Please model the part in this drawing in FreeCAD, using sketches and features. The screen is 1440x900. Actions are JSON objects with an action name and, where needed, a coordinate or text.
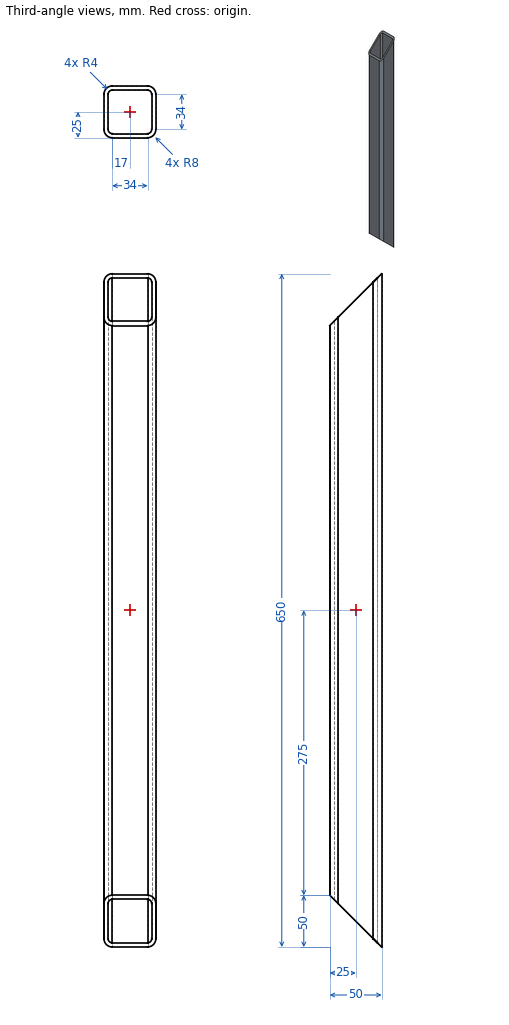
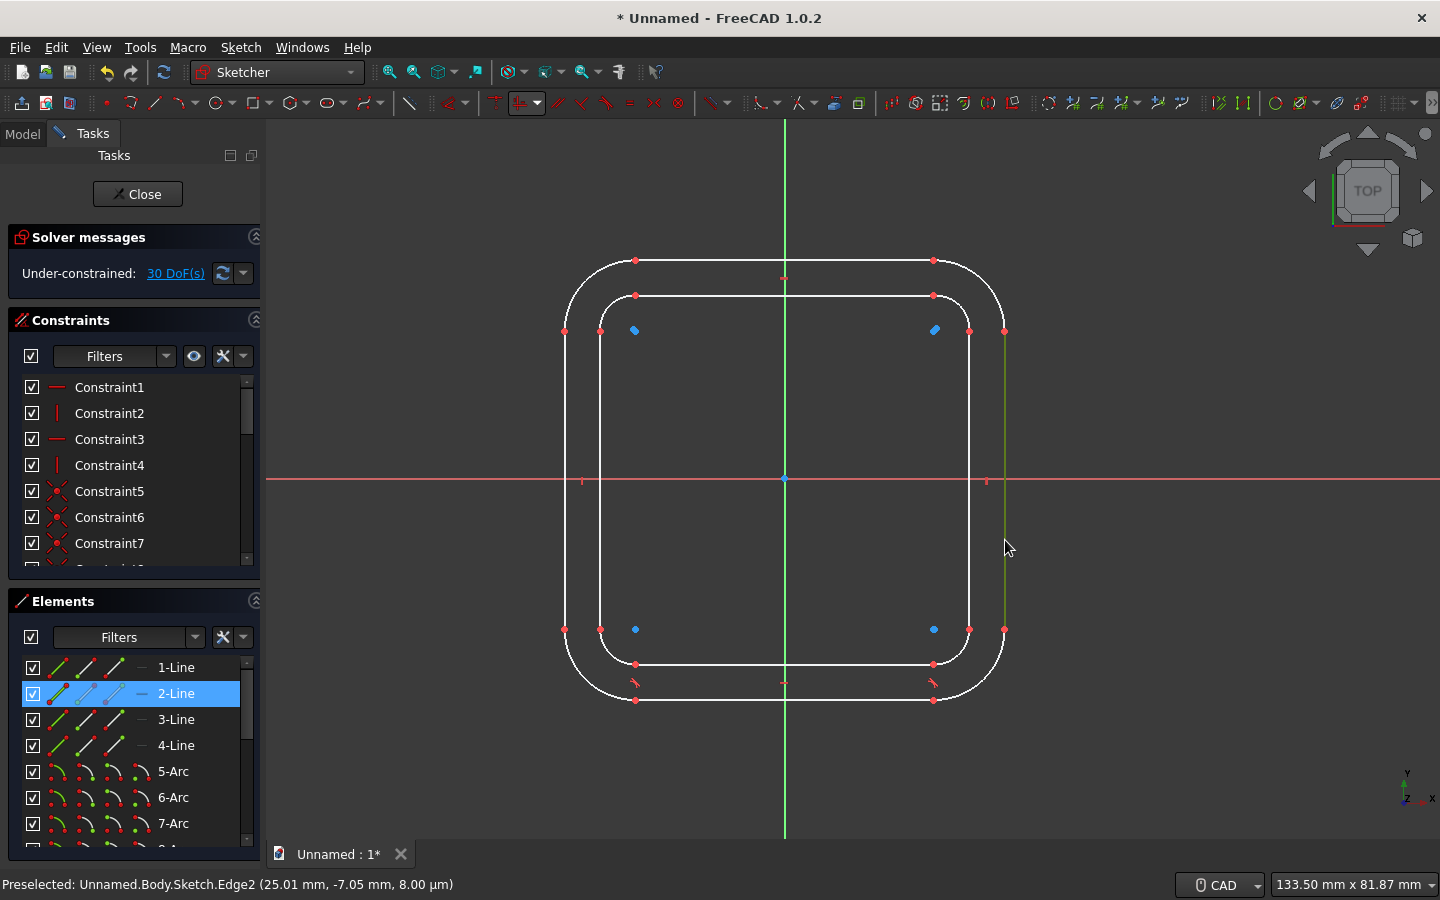
{"action": "left_click", "coordinate": [966, 692]}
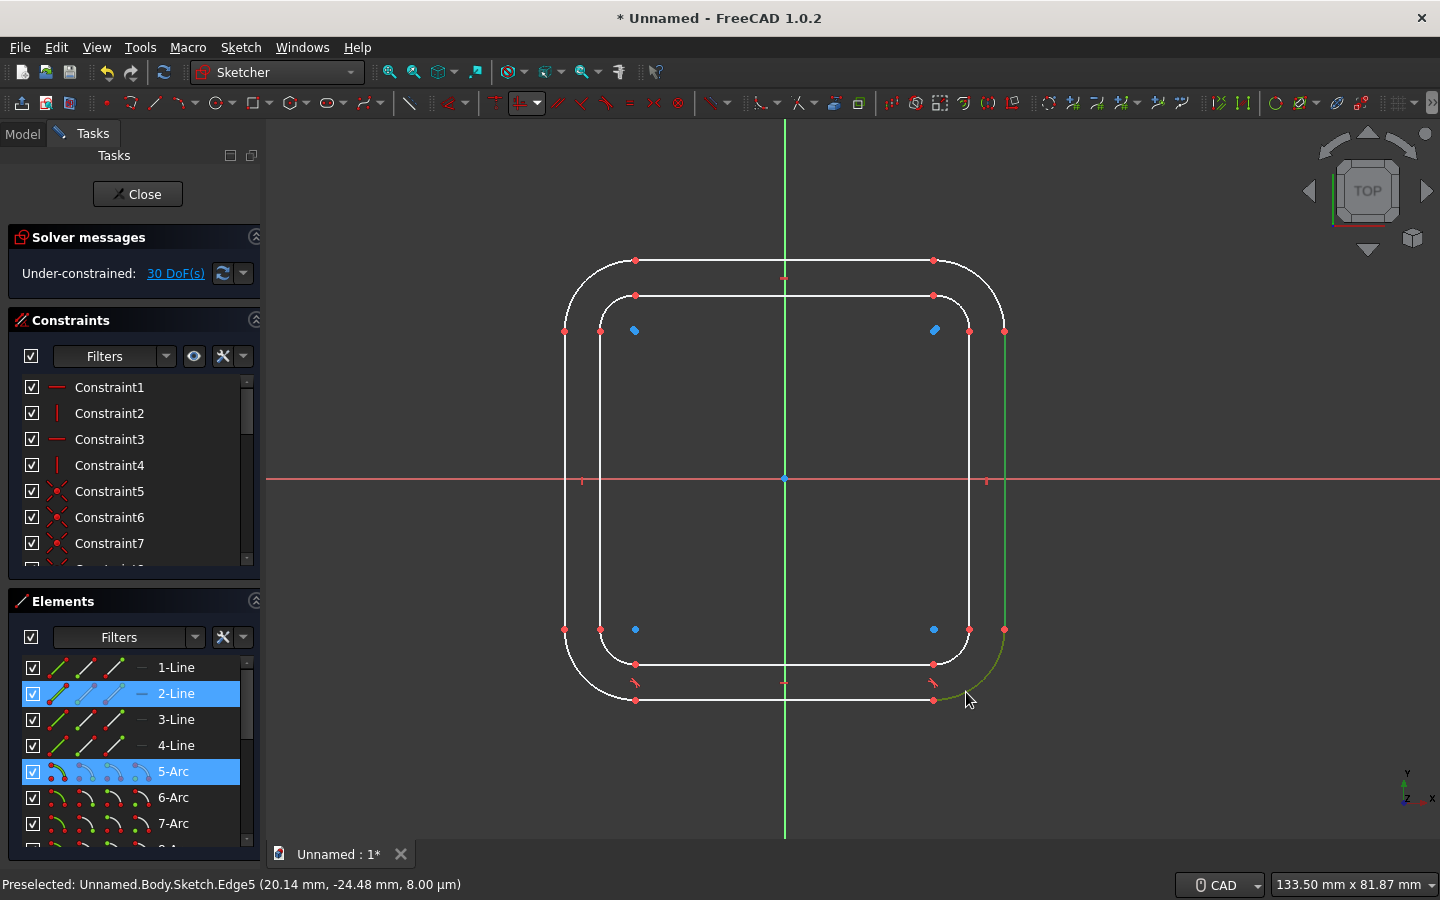
{"action": "left_click", "coordinate": [606, 104]}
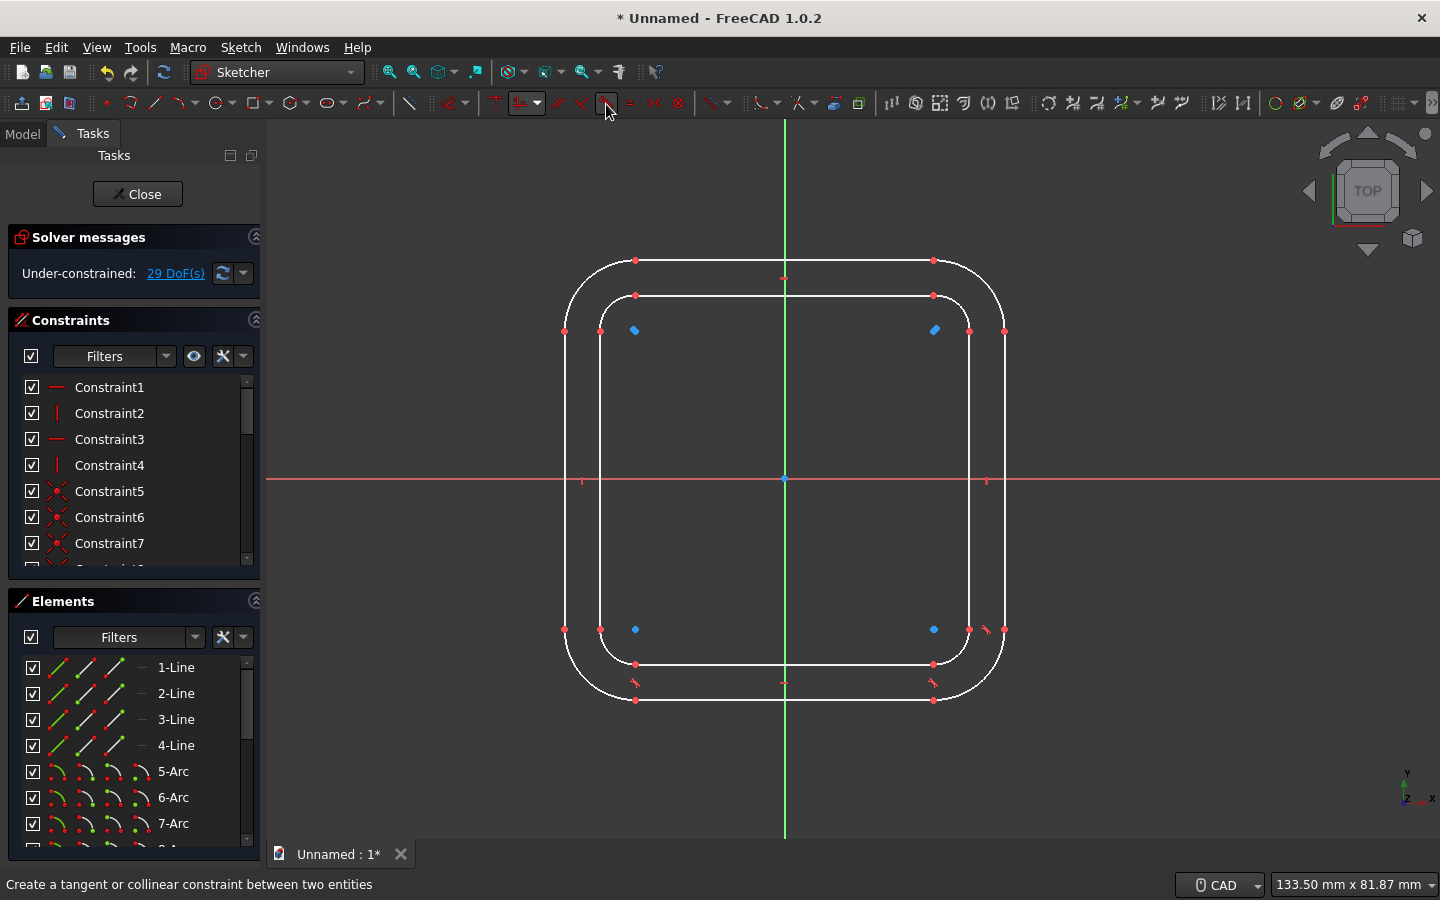
{"action": "left_click", "coordinate": [1005, 540]}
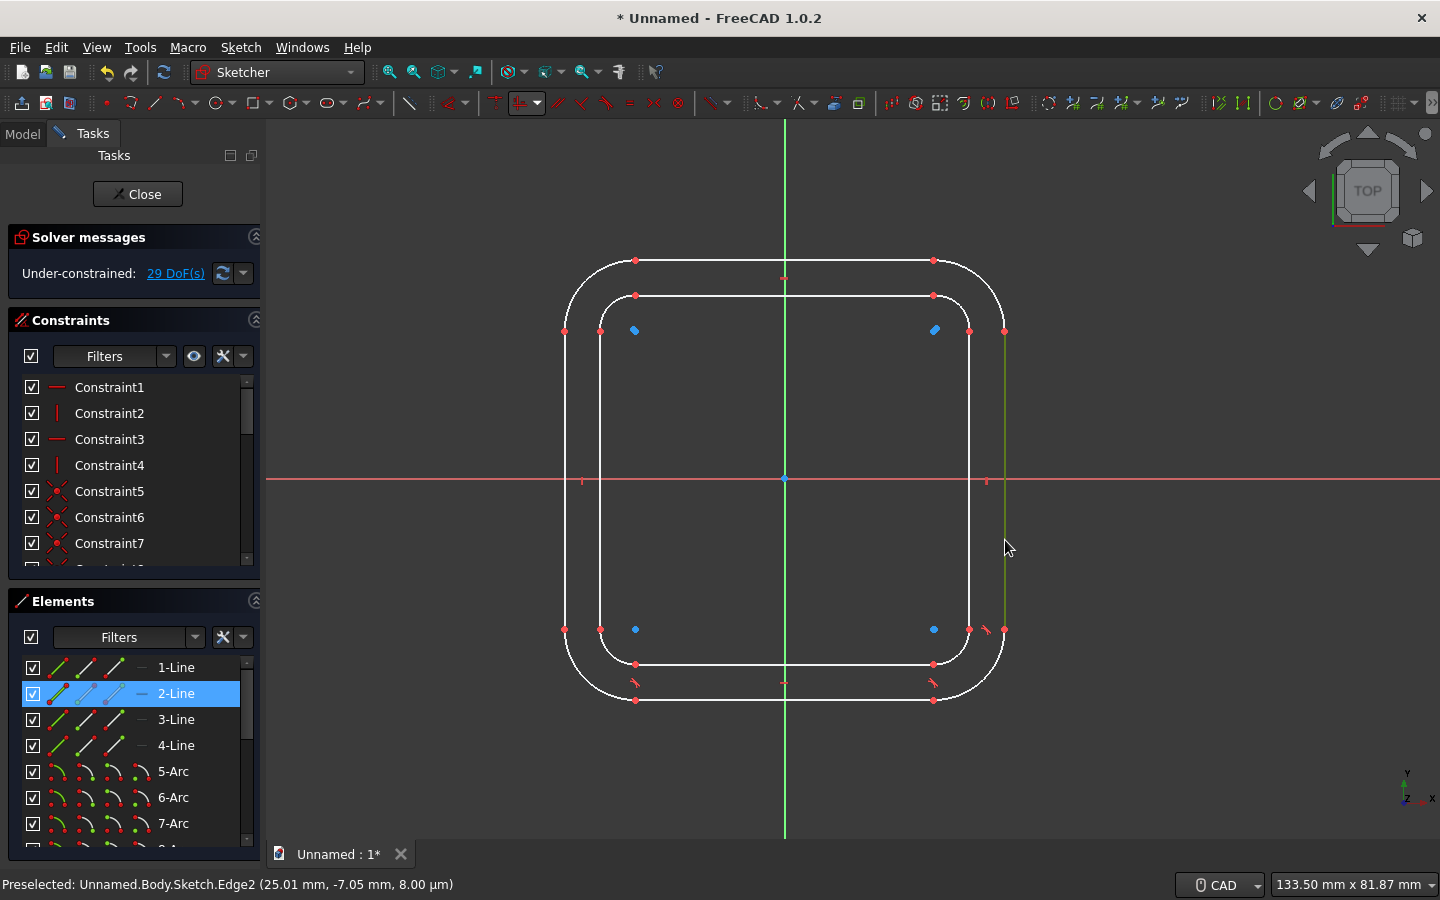
{"action": "left_click", "coordinate": [997, 299]}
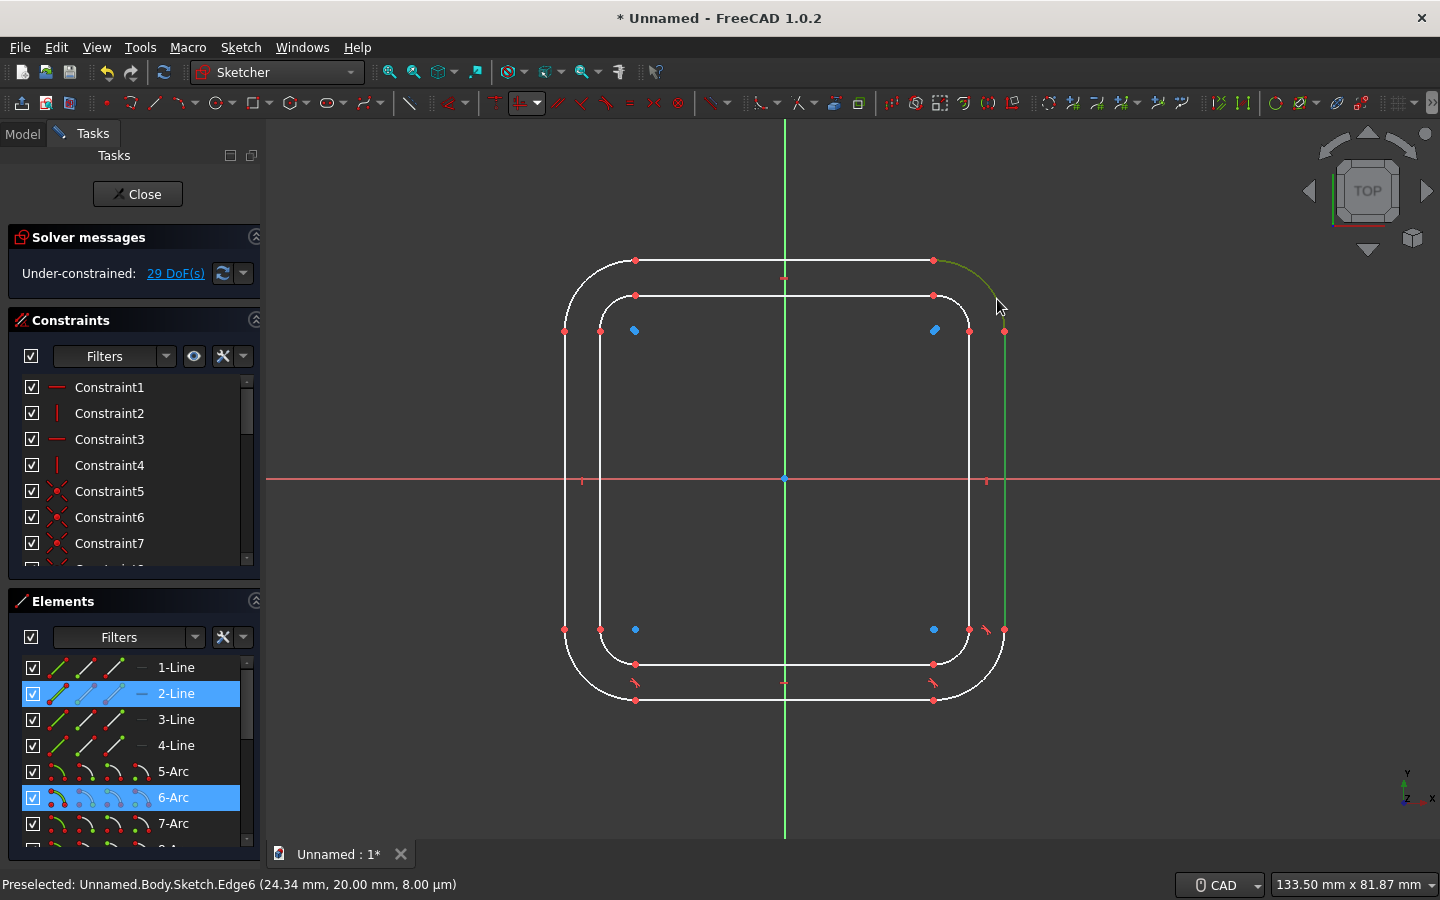
{"action": "left_click", "coordinate": [606, 104]}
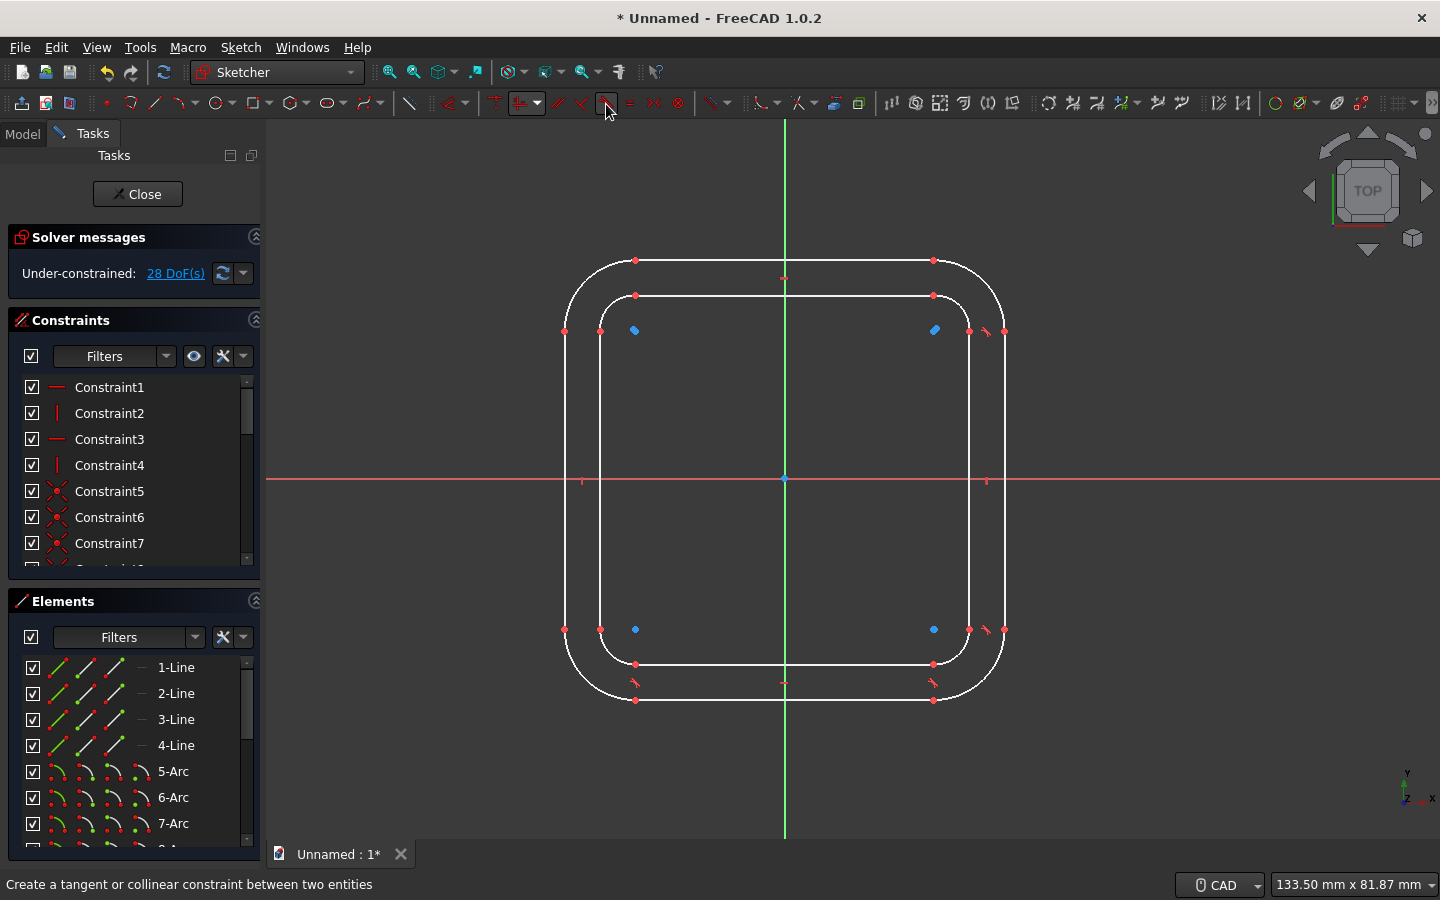
{"action": "left_click", "coordinate": [844, 260]}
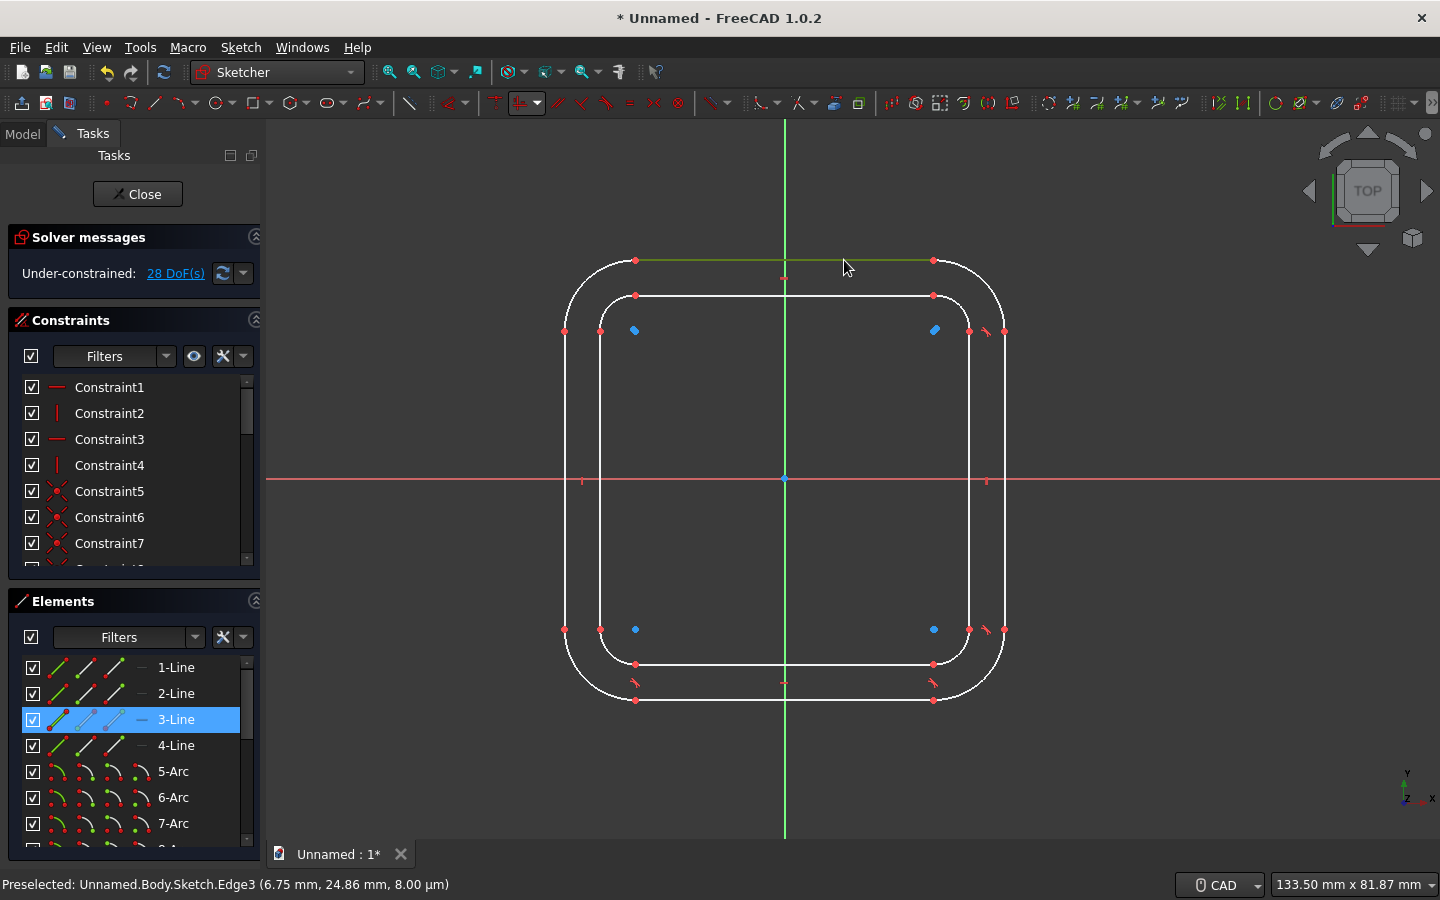
{"action": "left_click", "coordinate": [997, 299]}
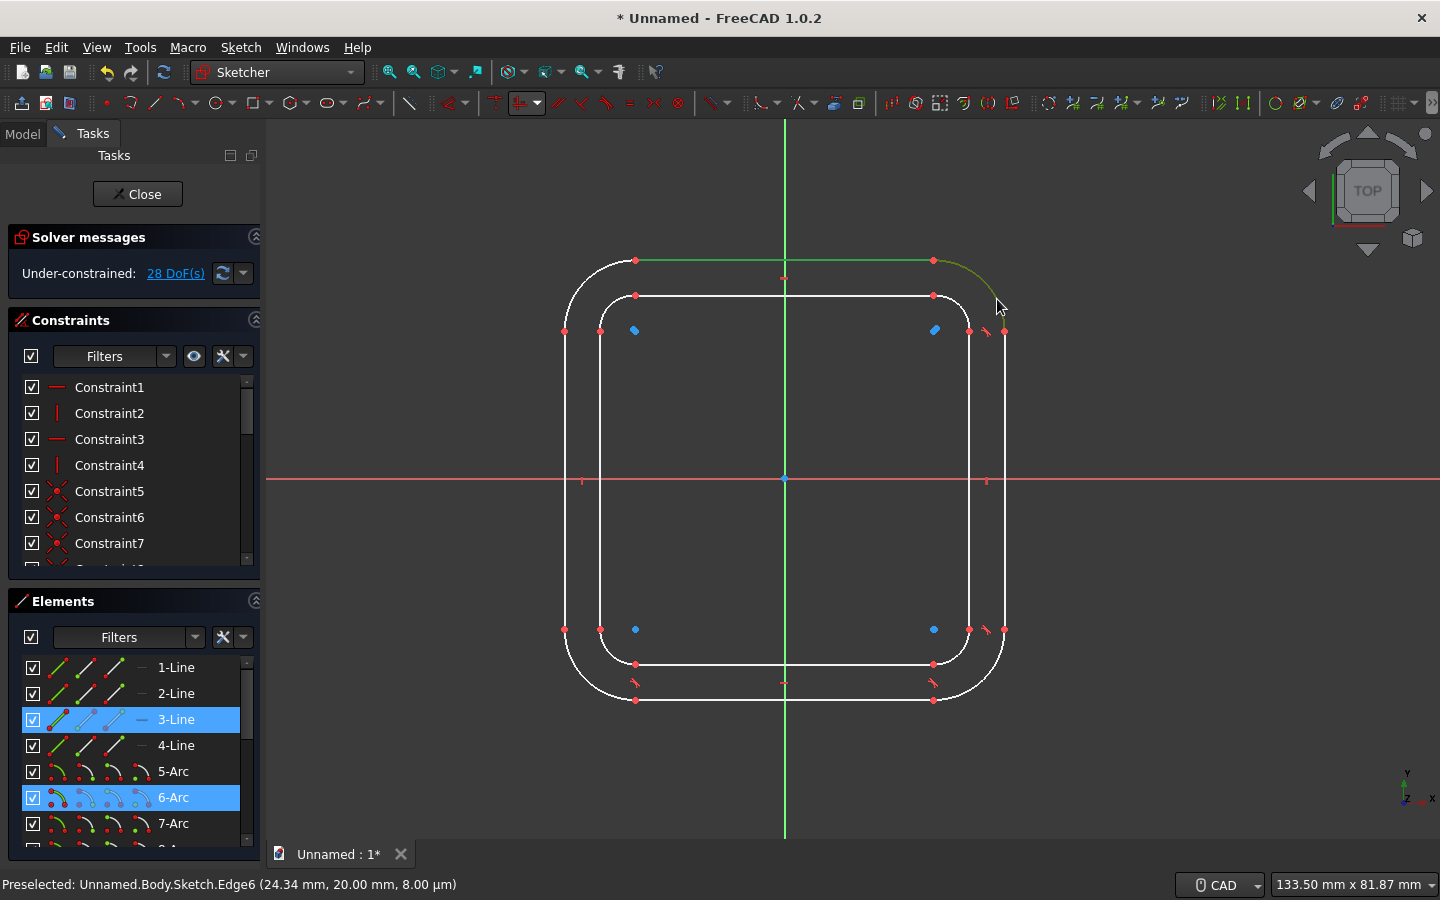
{"action": "left_click", "coordinate": [606, 104]}